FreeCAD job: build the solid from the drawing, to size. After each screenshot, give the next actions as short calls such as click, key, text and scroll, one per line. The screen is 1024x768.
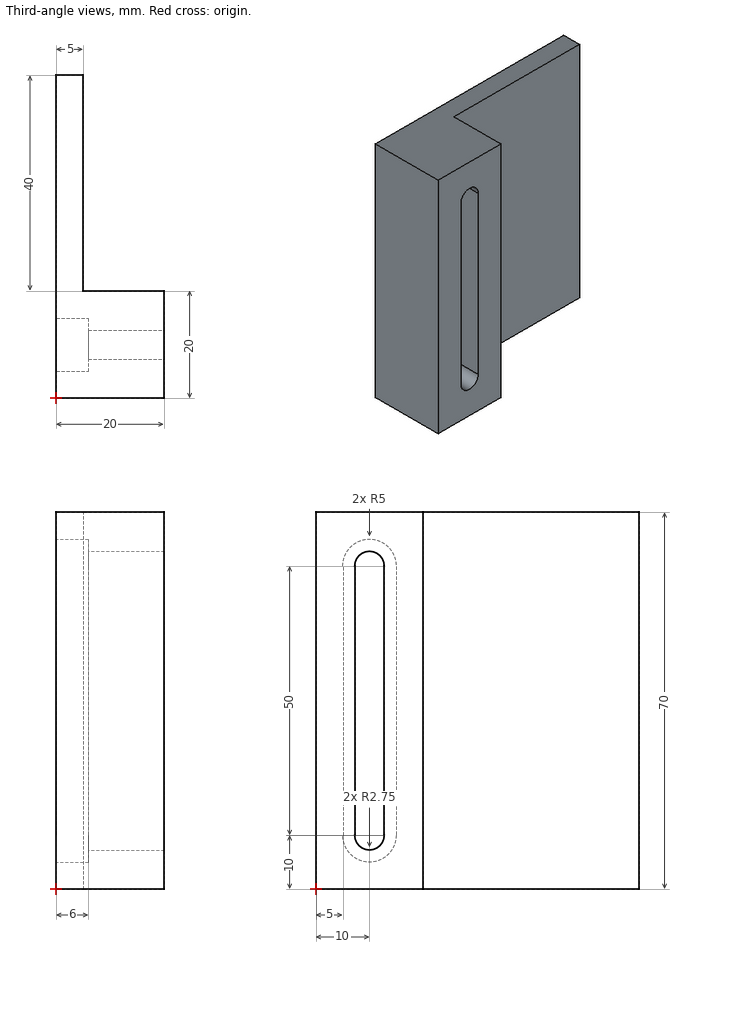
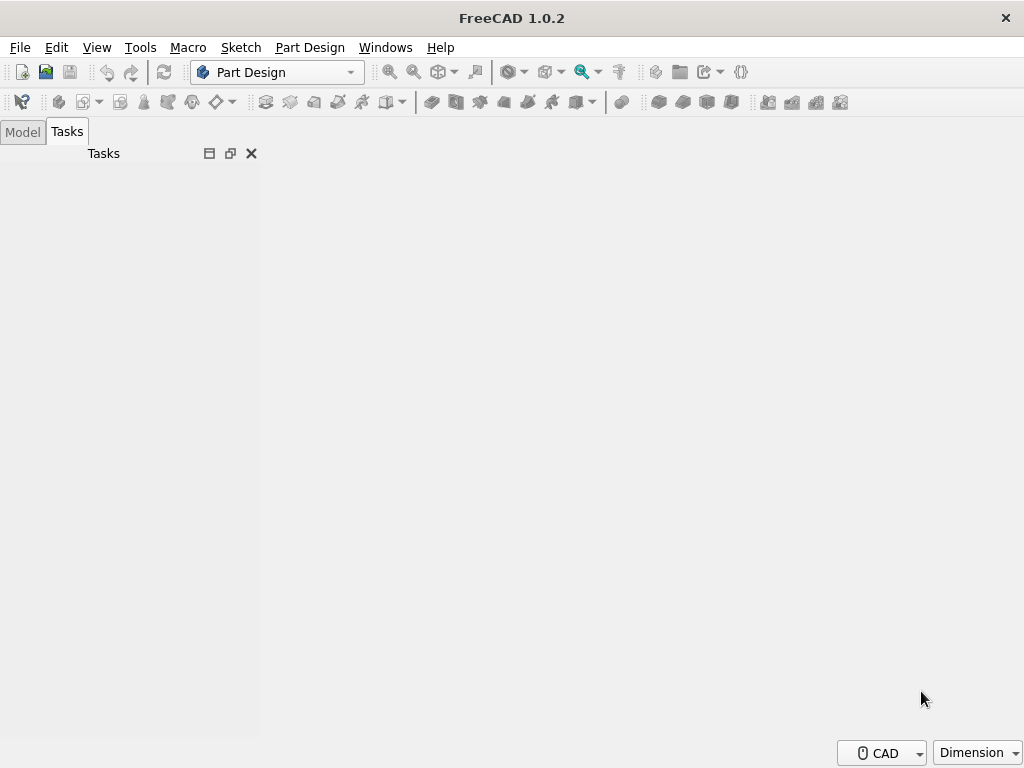
click(22, 72)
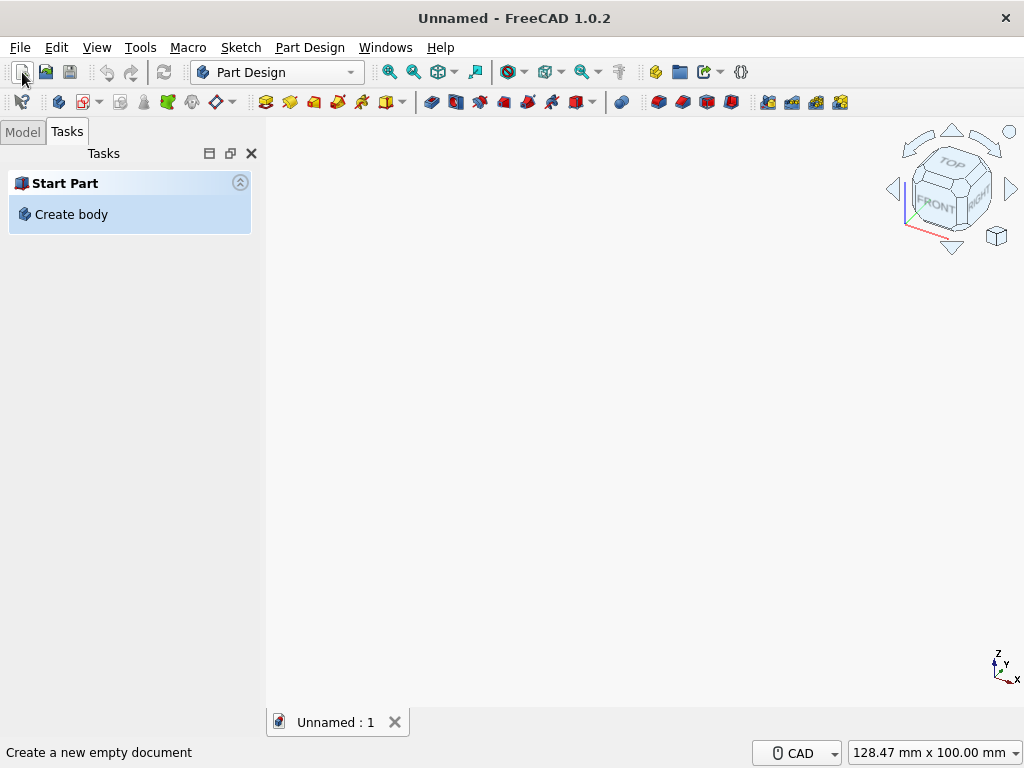
click(84, 102)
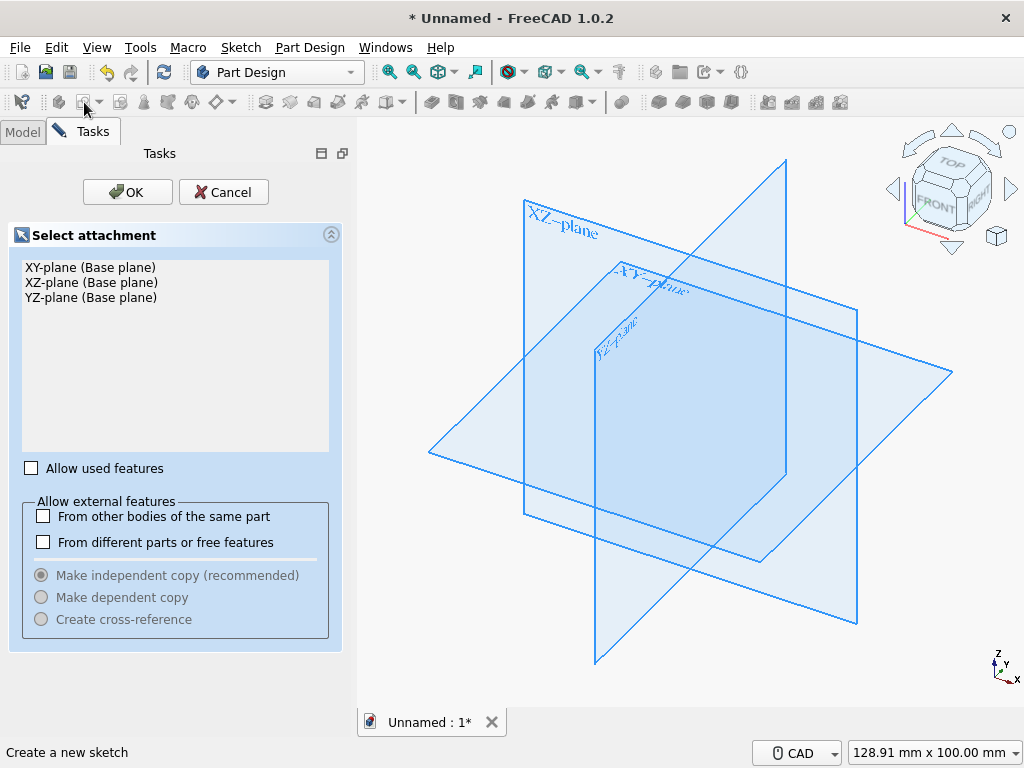
click(82, 268)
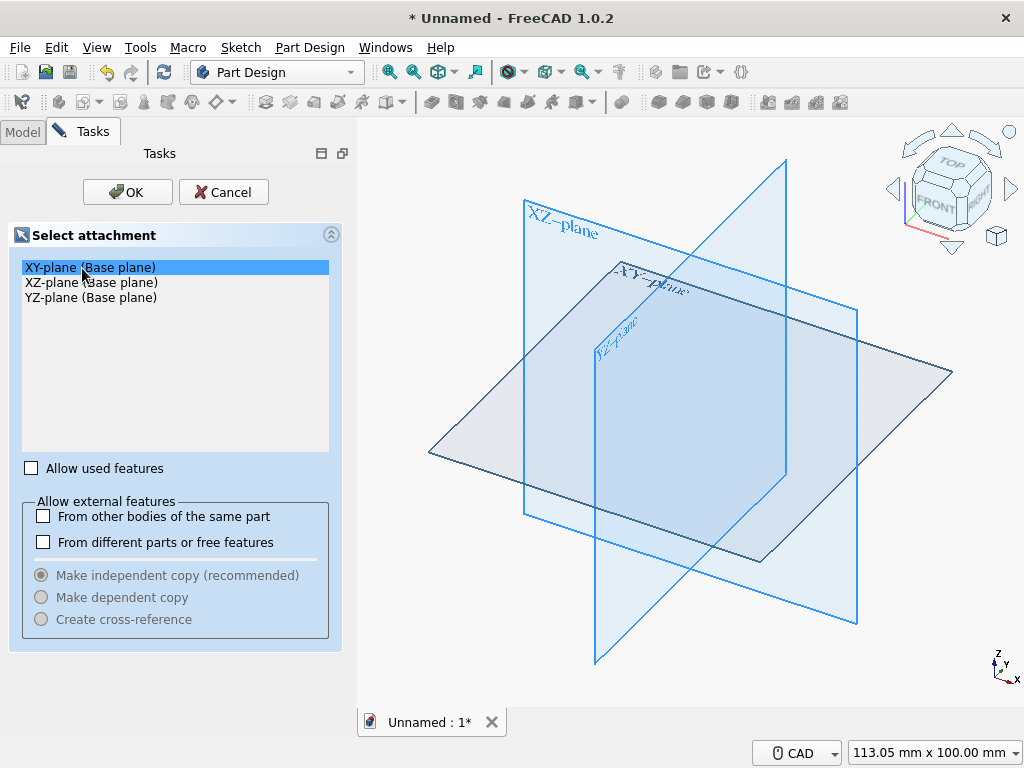
click(128, 192)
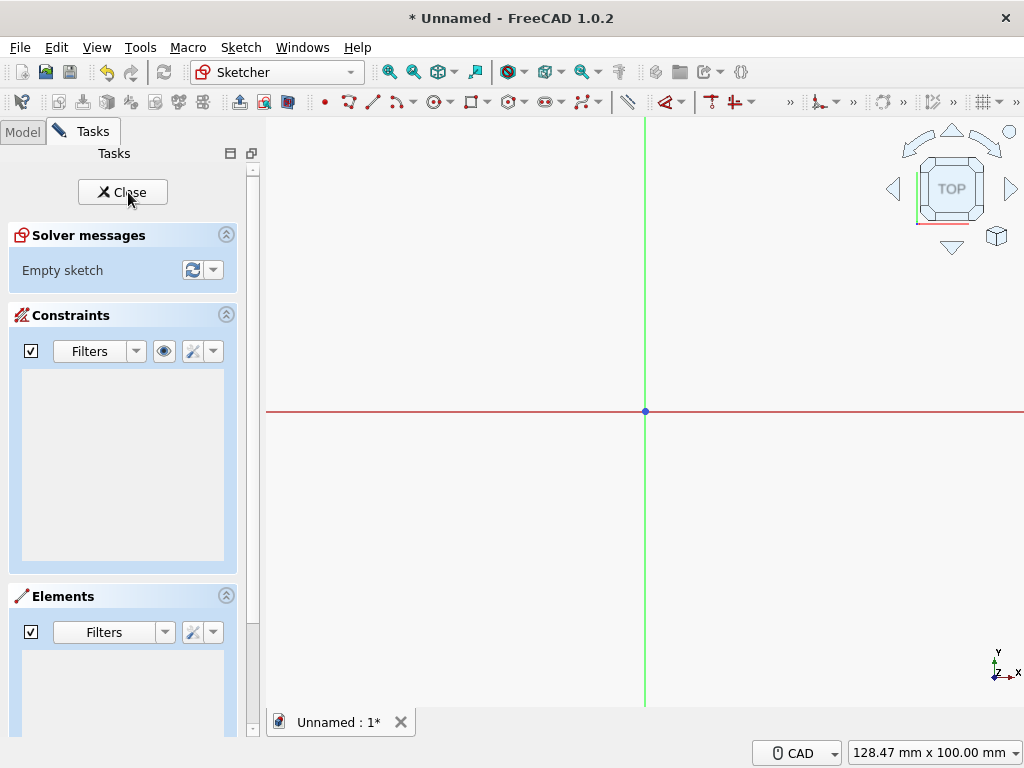
scroll(294, 679, down, 1)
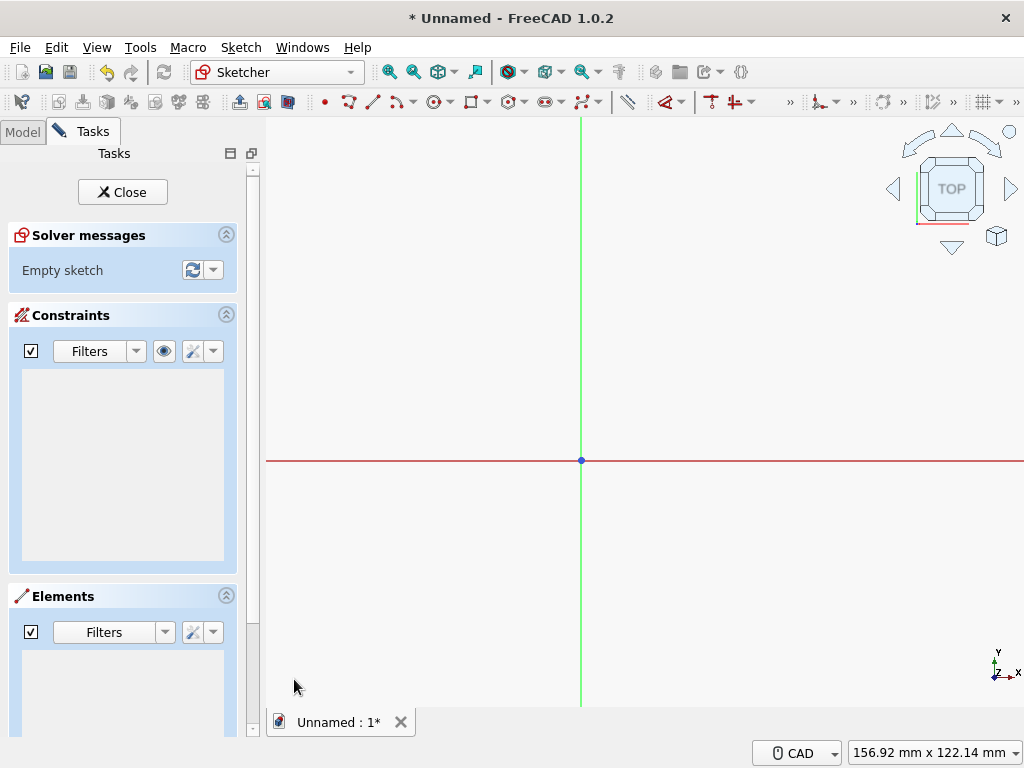
click(350, 102)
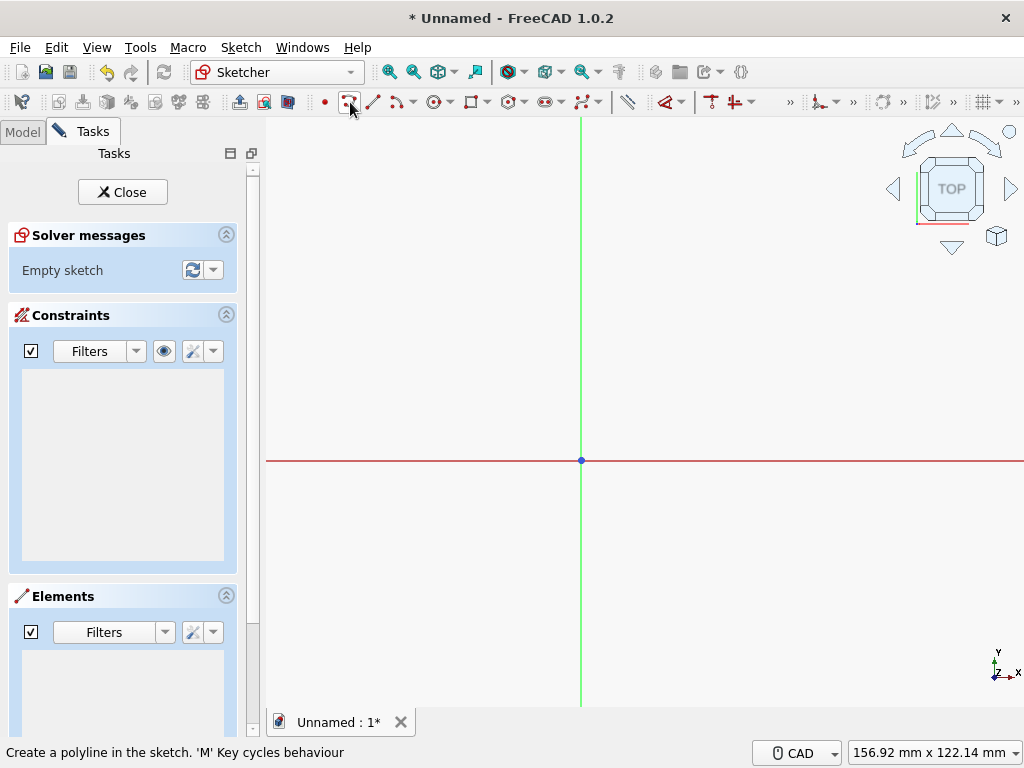
click(581, 461)
click(678, 452)
click(678, 364)
click(606, 364)
click(606, 171)
click(590, 171)
click(581, 461)
key(Escape)
key(Escape)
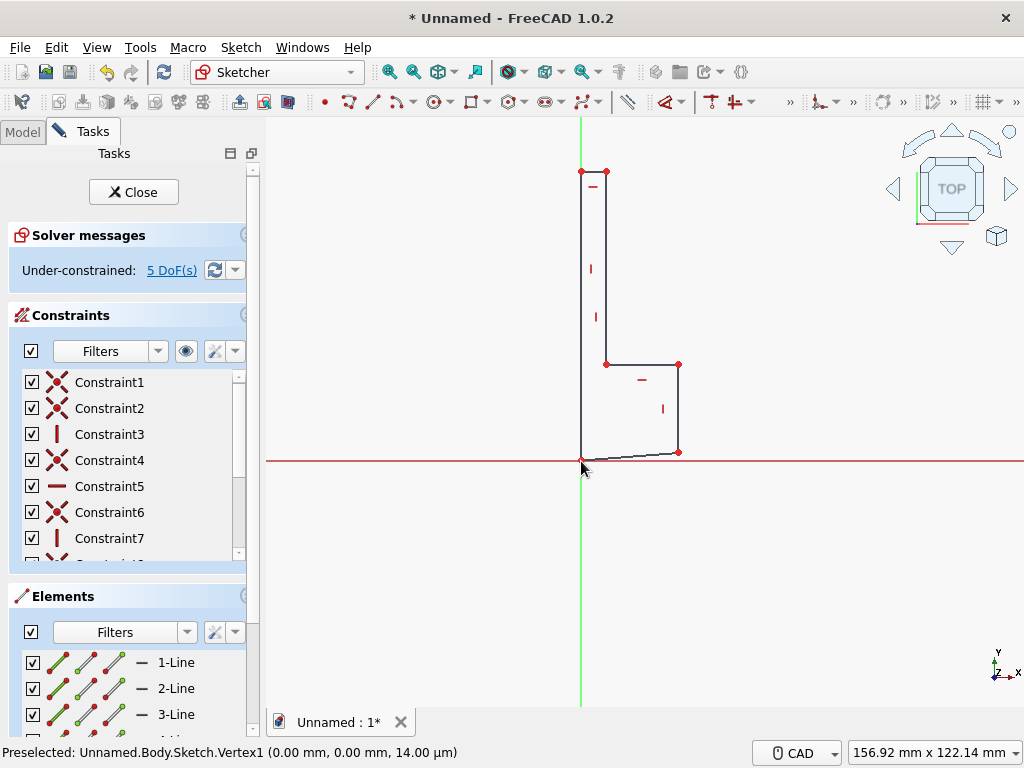
click(610, 458)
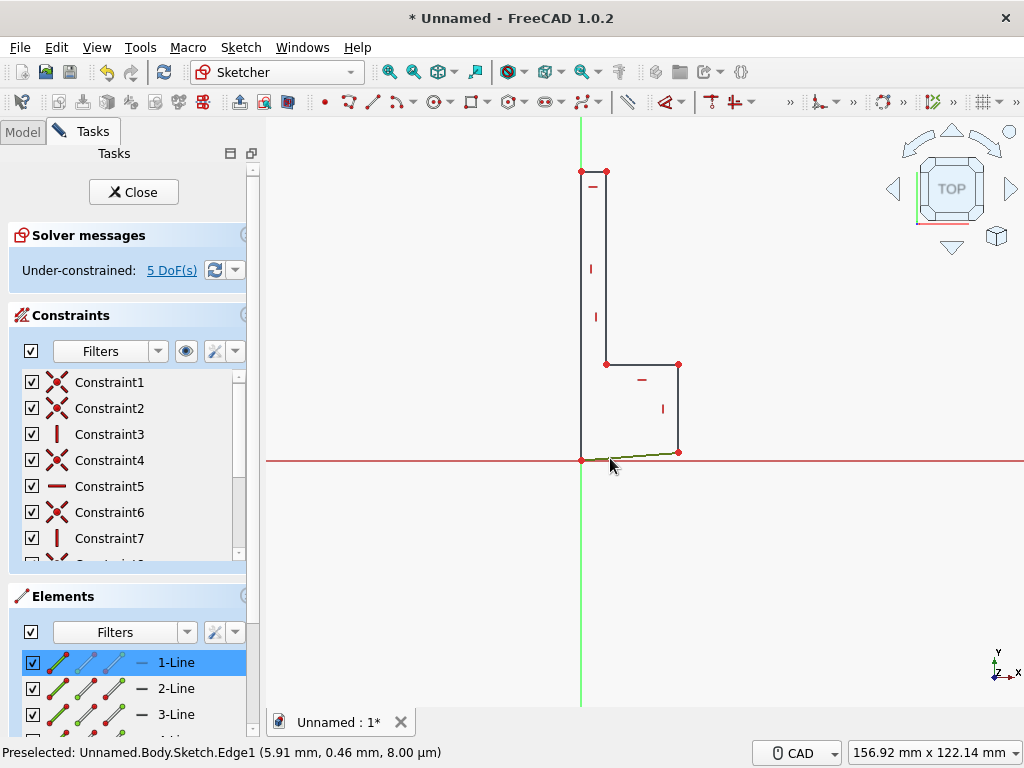
key(h)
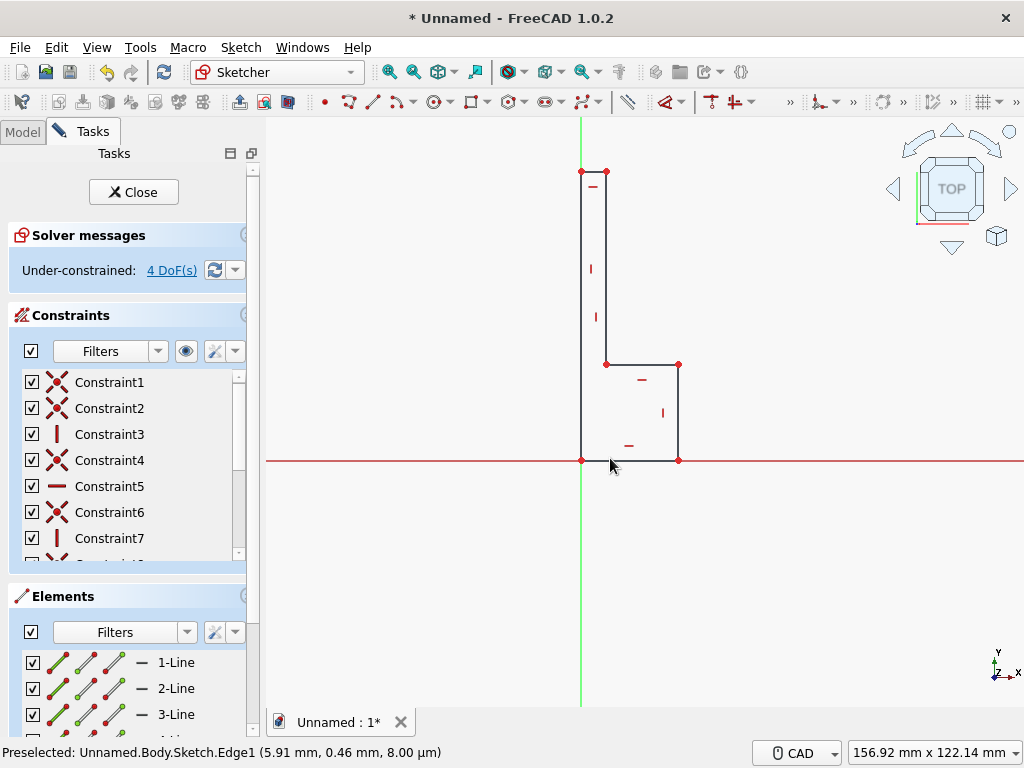
click(666, 102)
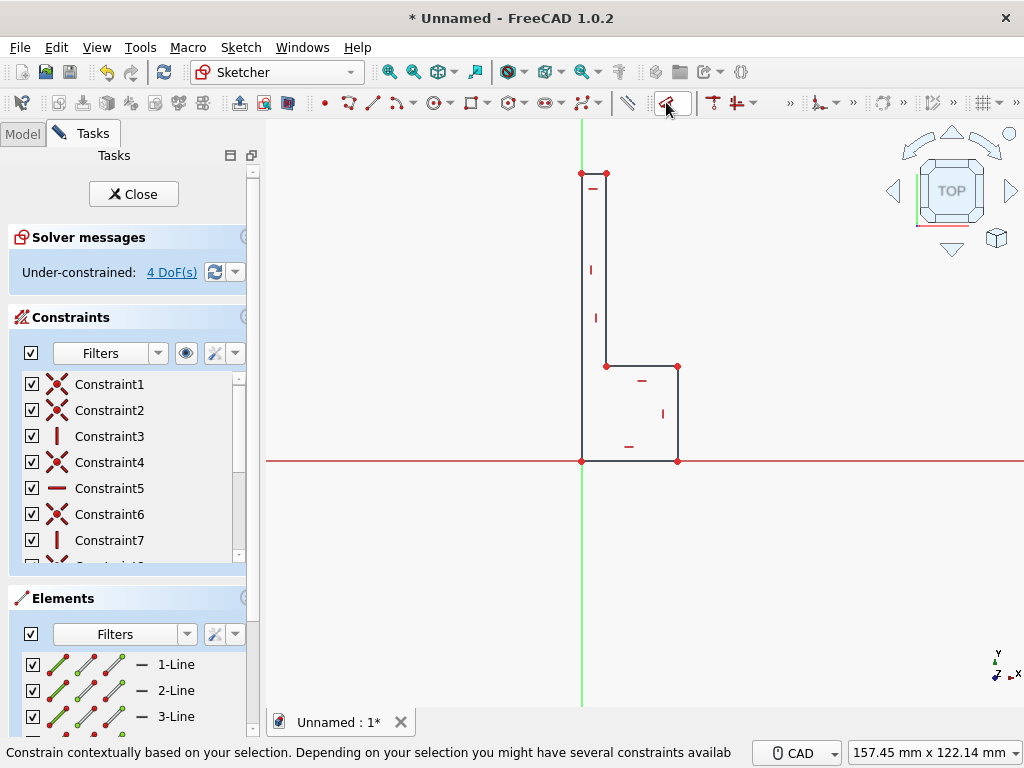
scroll(596, 174, up, 3)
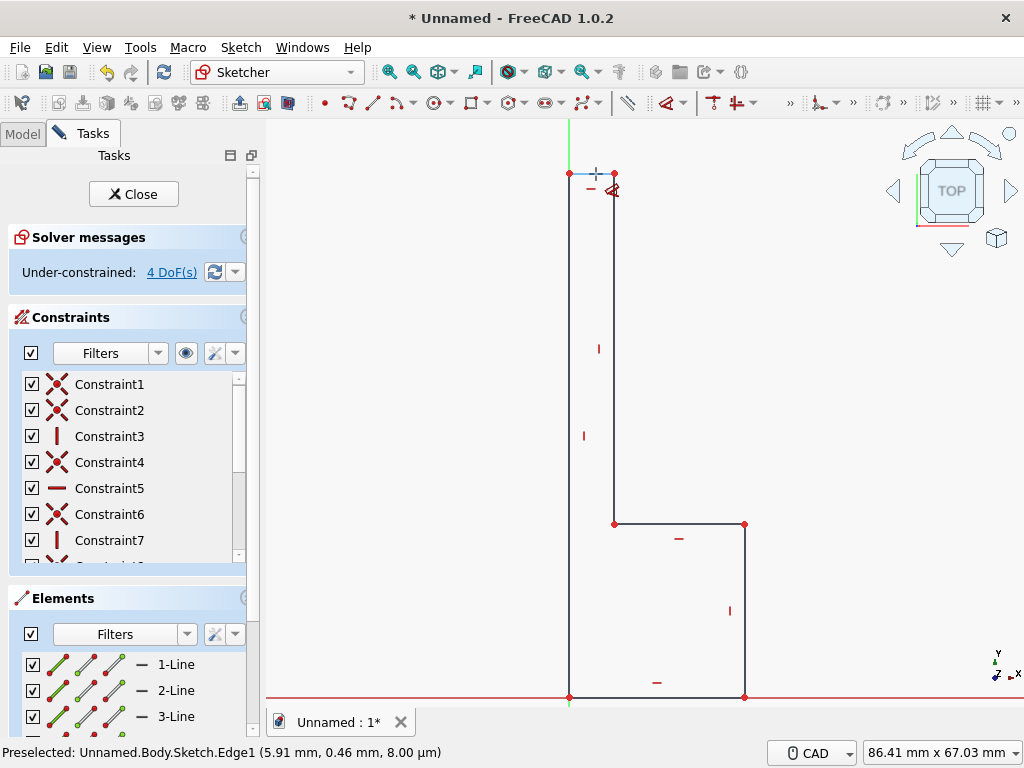
click(596, 174)
click(592, 208)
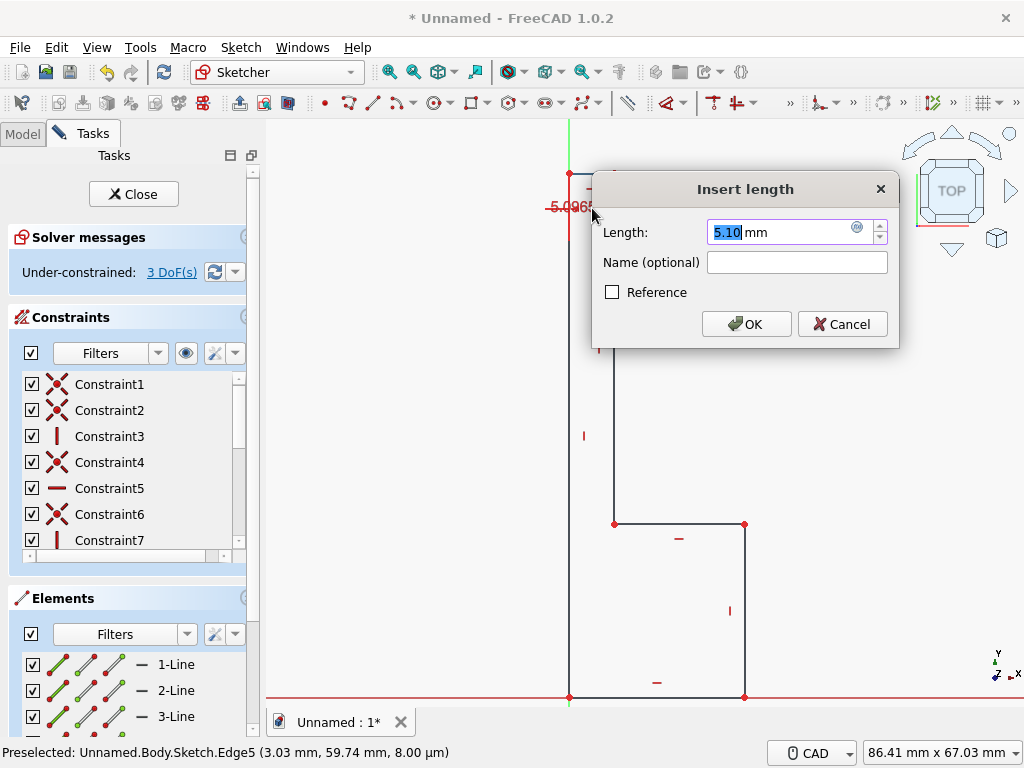
text(5)
key(Return)